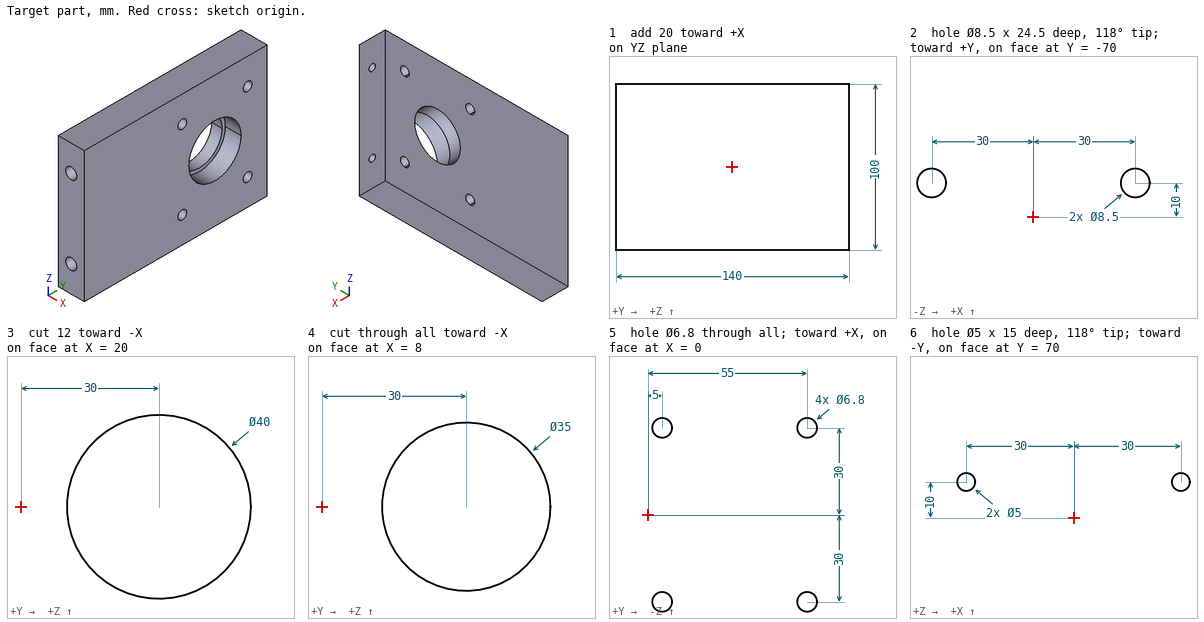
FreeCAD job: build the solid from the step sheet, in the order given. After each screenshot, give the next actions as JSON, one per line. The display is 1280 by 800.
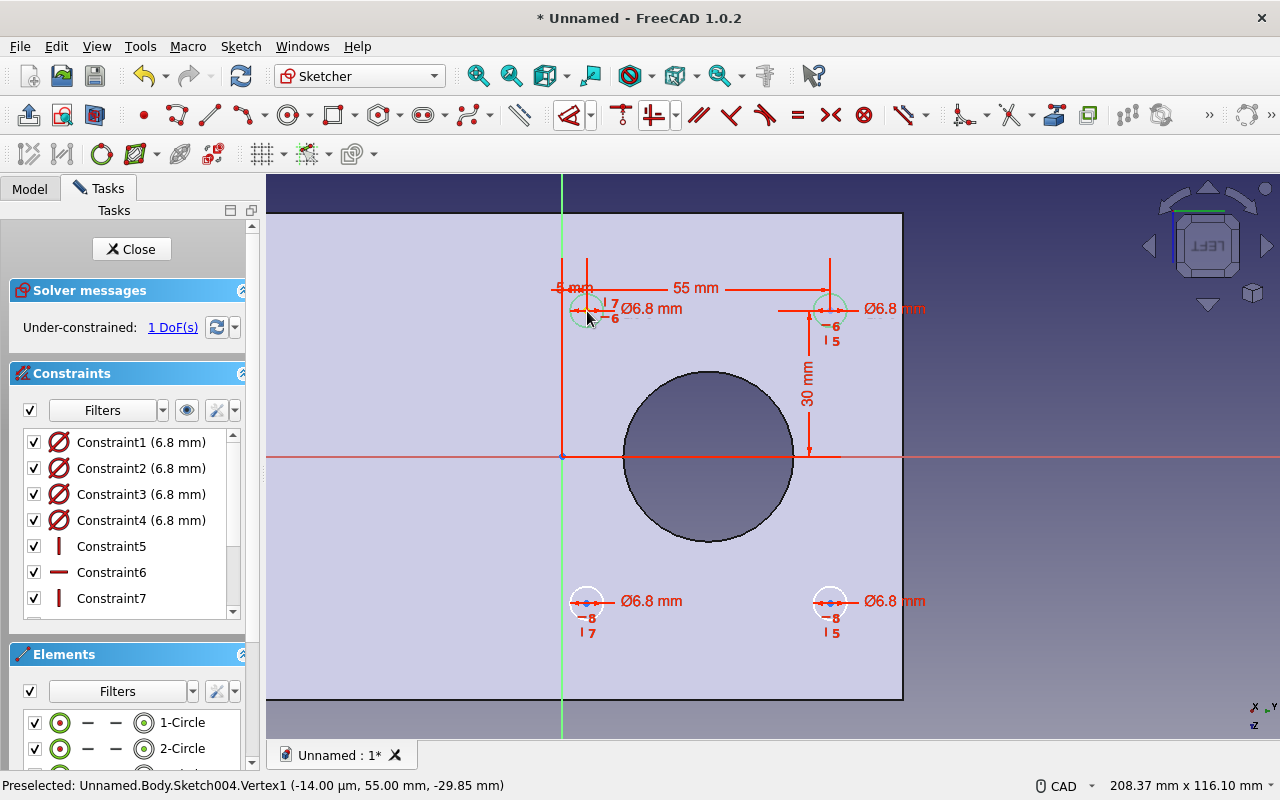
{"action": "left_click", "coordinate": [830, 603]}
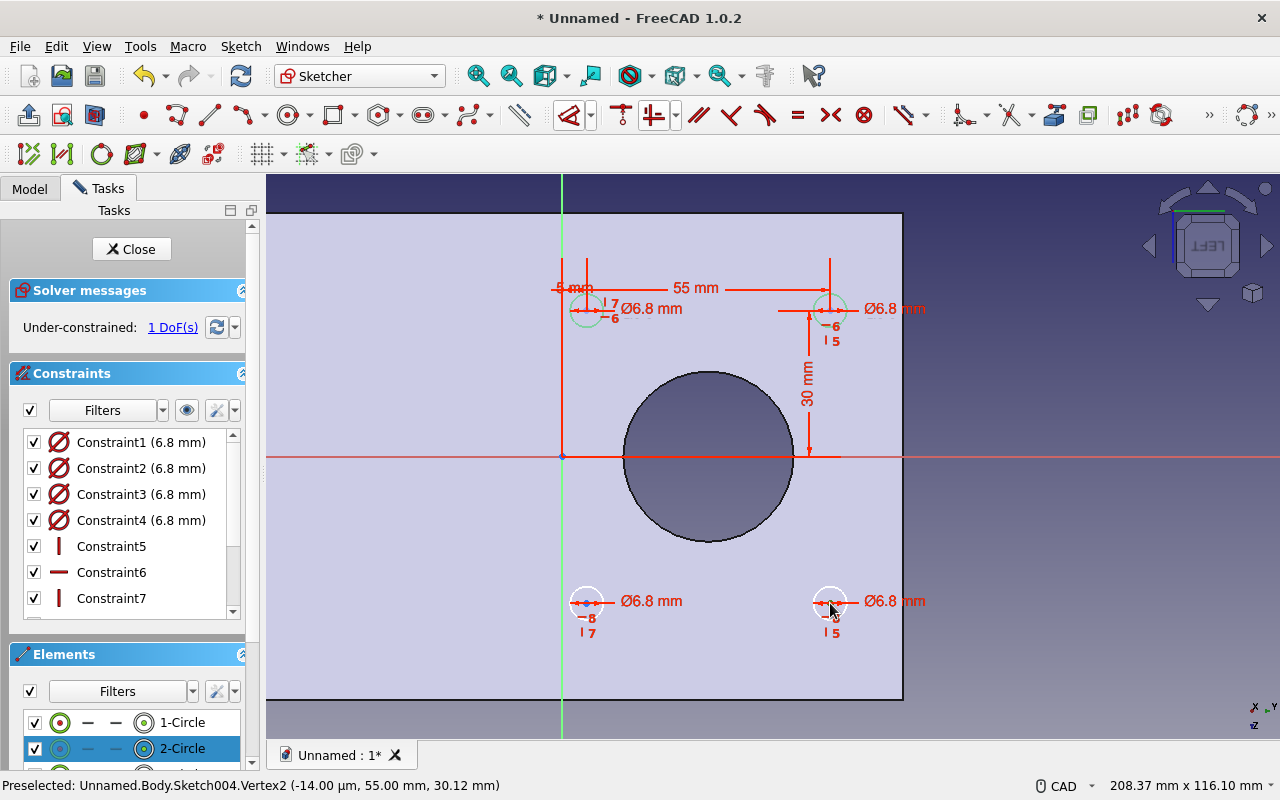
{"action": "key", "text": "i"}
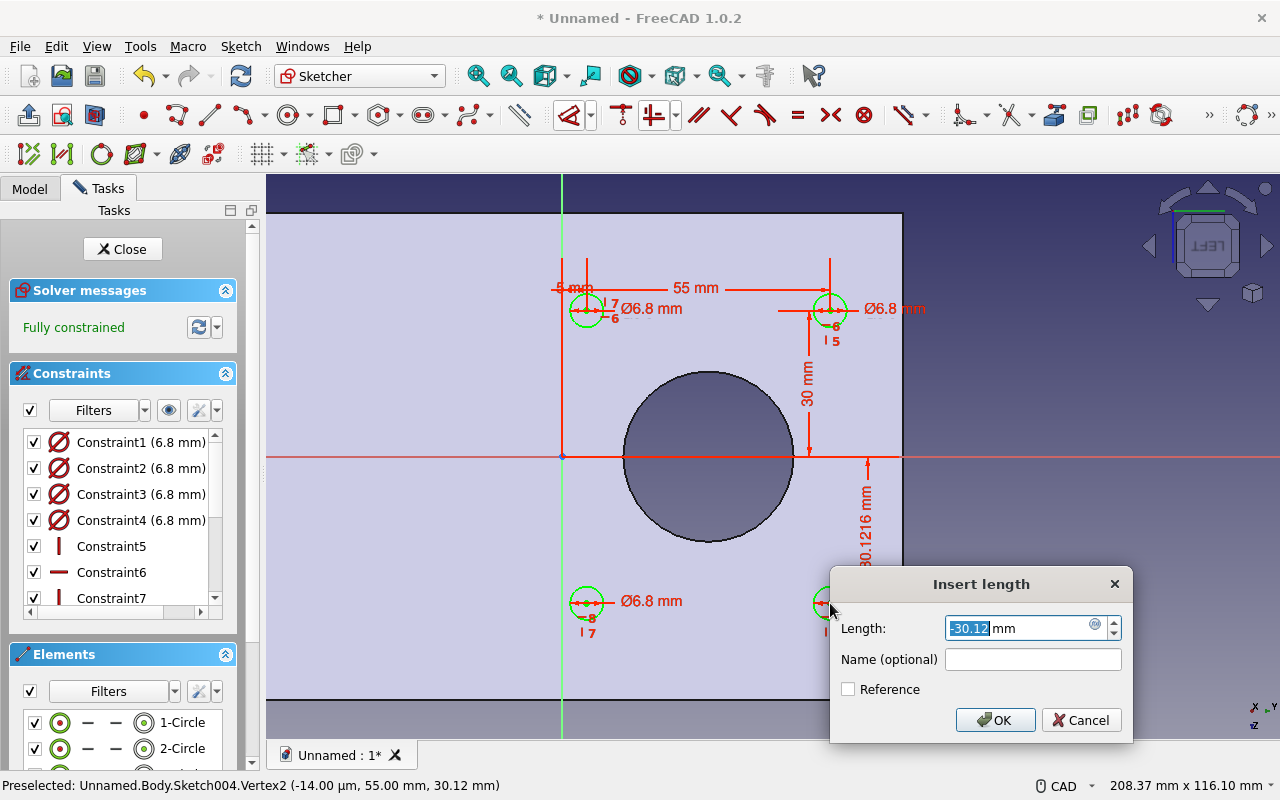
{"action": "type", "text": "-30"}
{"action": "key", "text": "Return"}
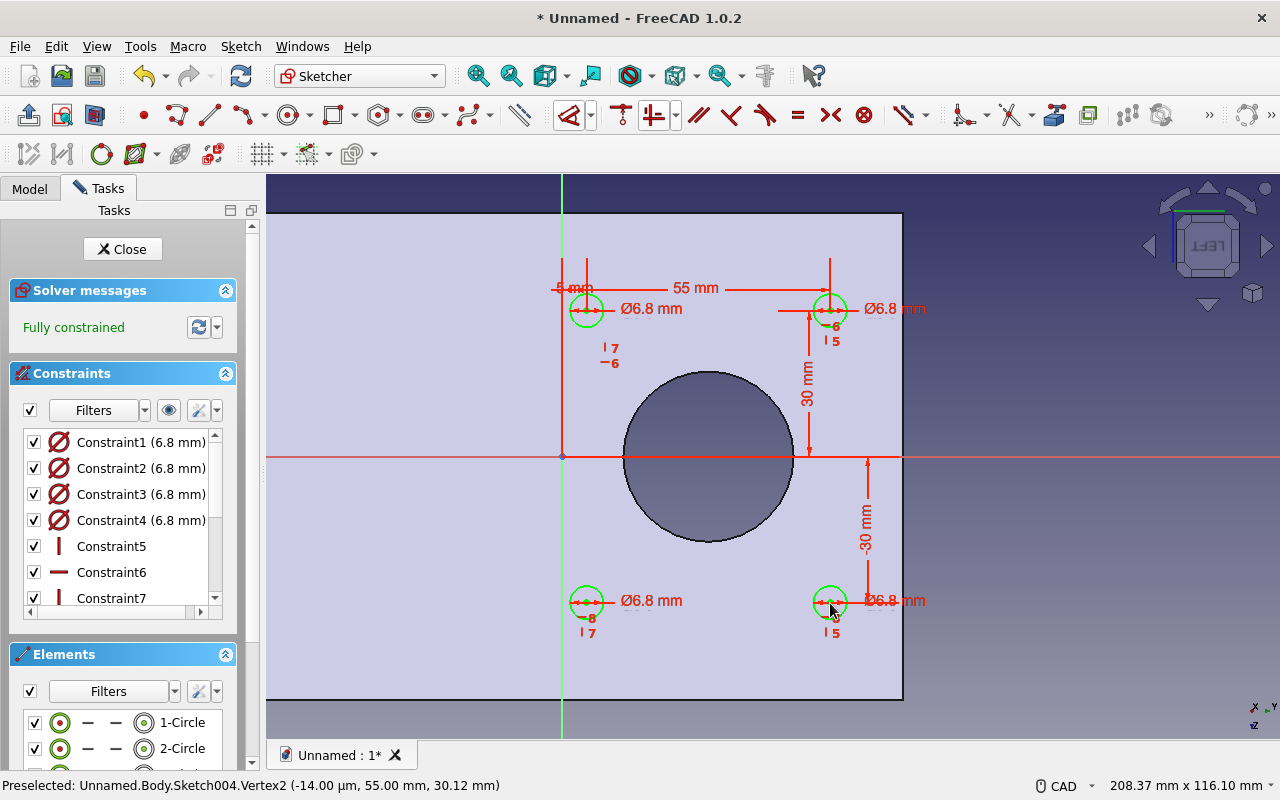
{"action": "left_click", "coordinate": [123, 249]}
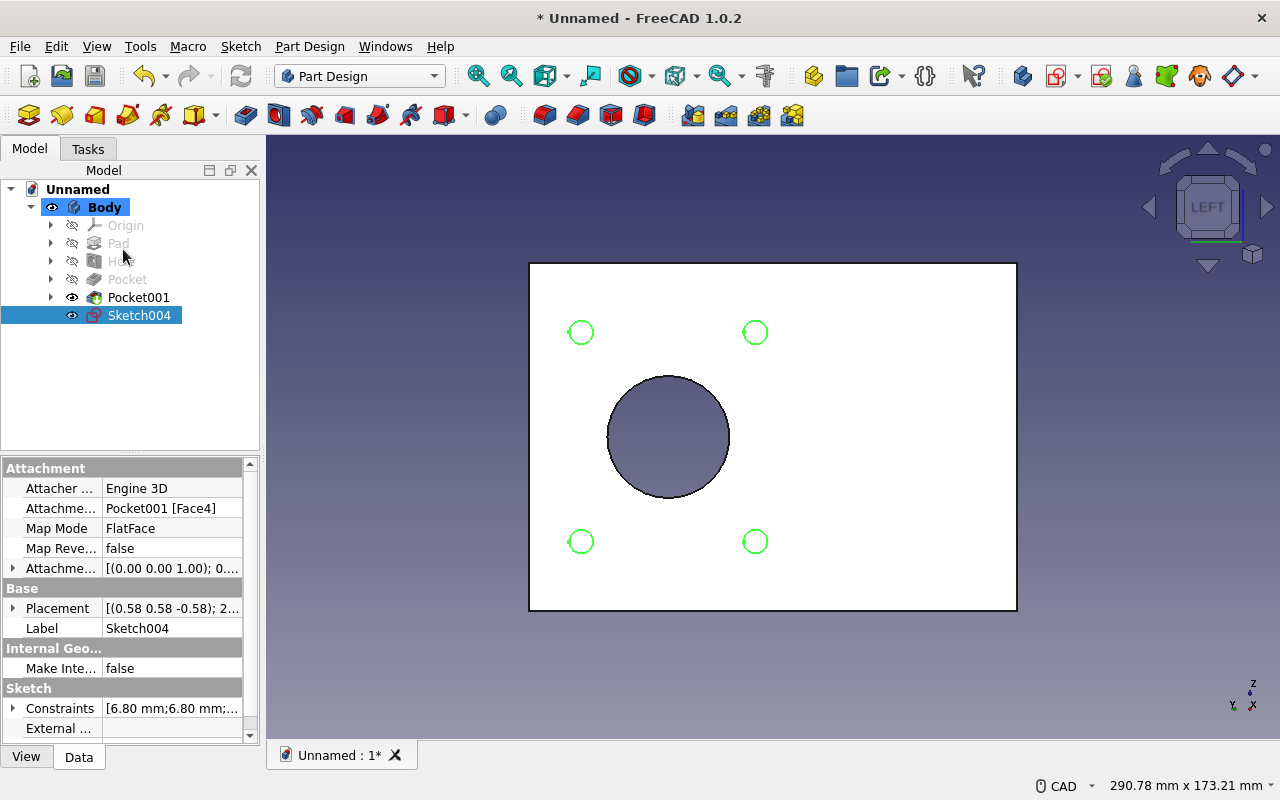
{"action": "left_click", "coordinate": [279, 116]}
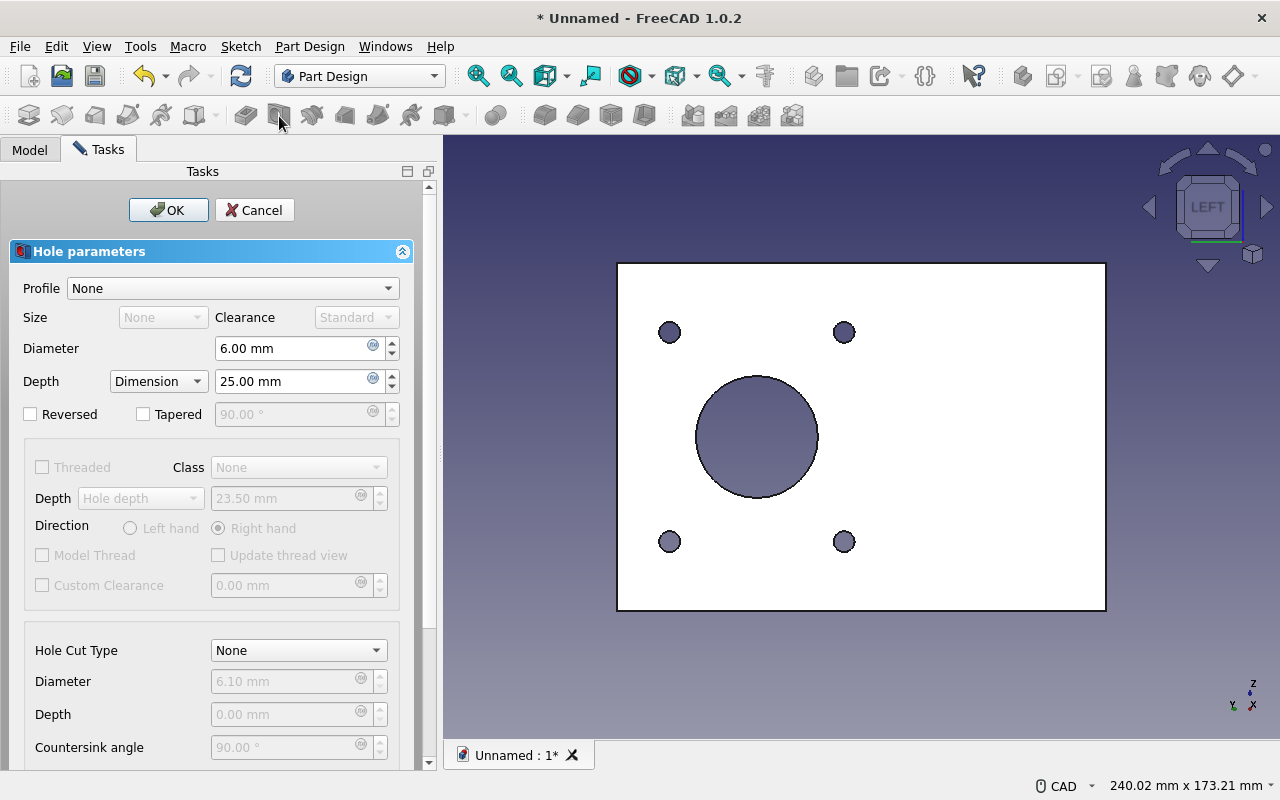
{"action": "triple_click", "coordinate": [300, 348]}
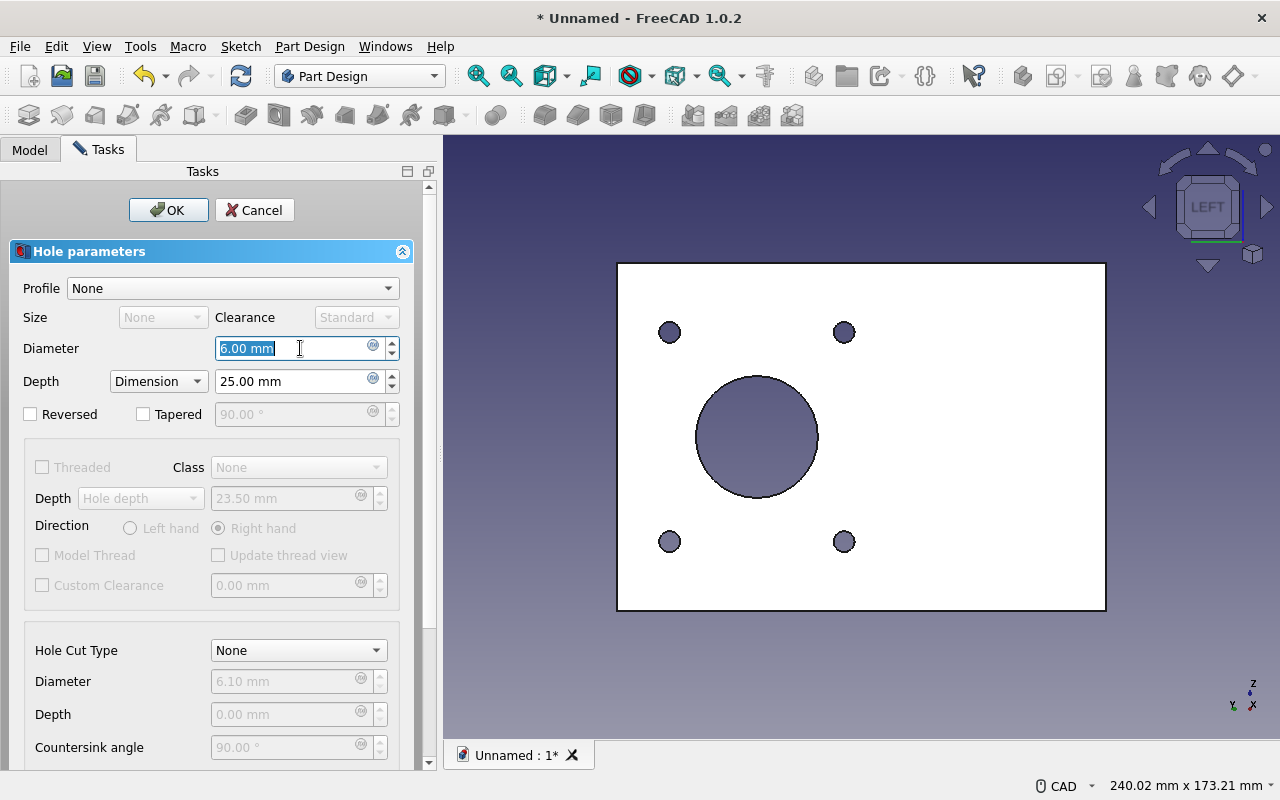
{"action": "type", "text": "6.8"}
{"action": "key", "text": "Tab"}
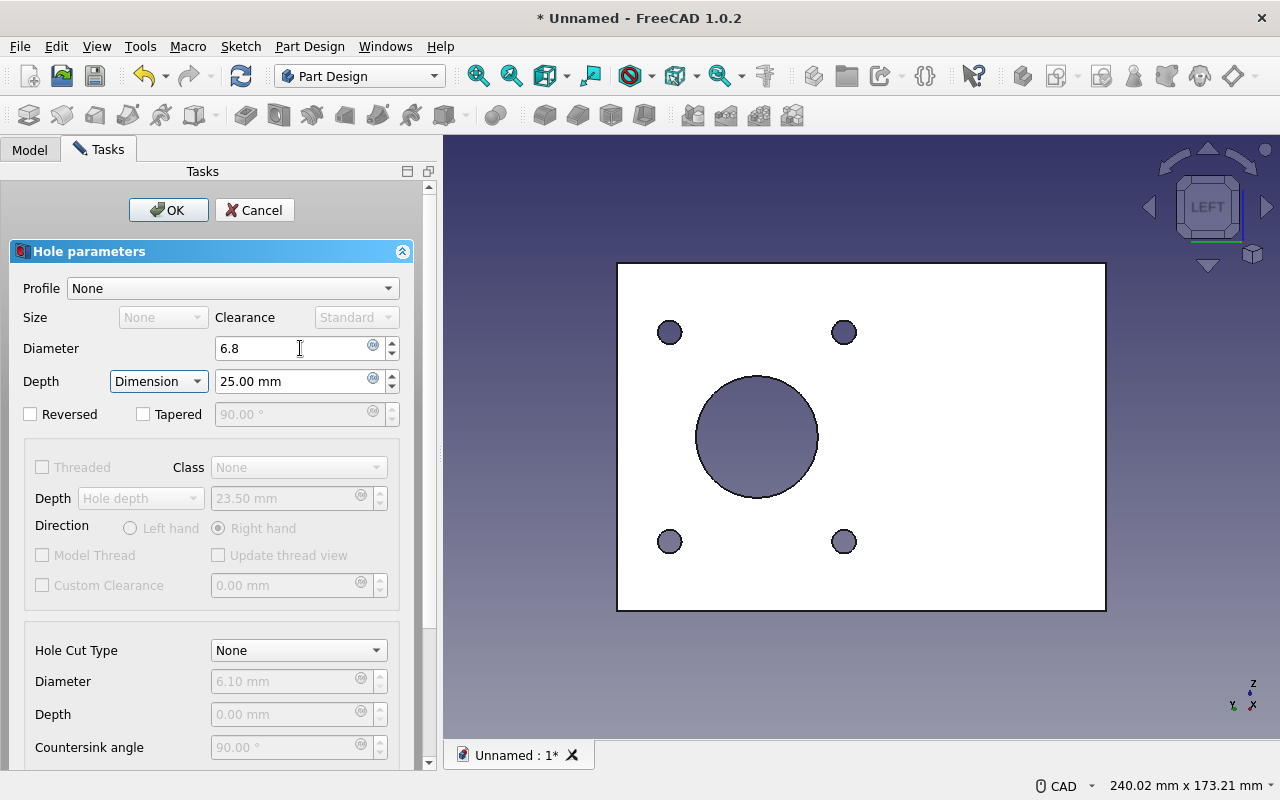
{"action": "left_click", "coordinate": [160, 382]}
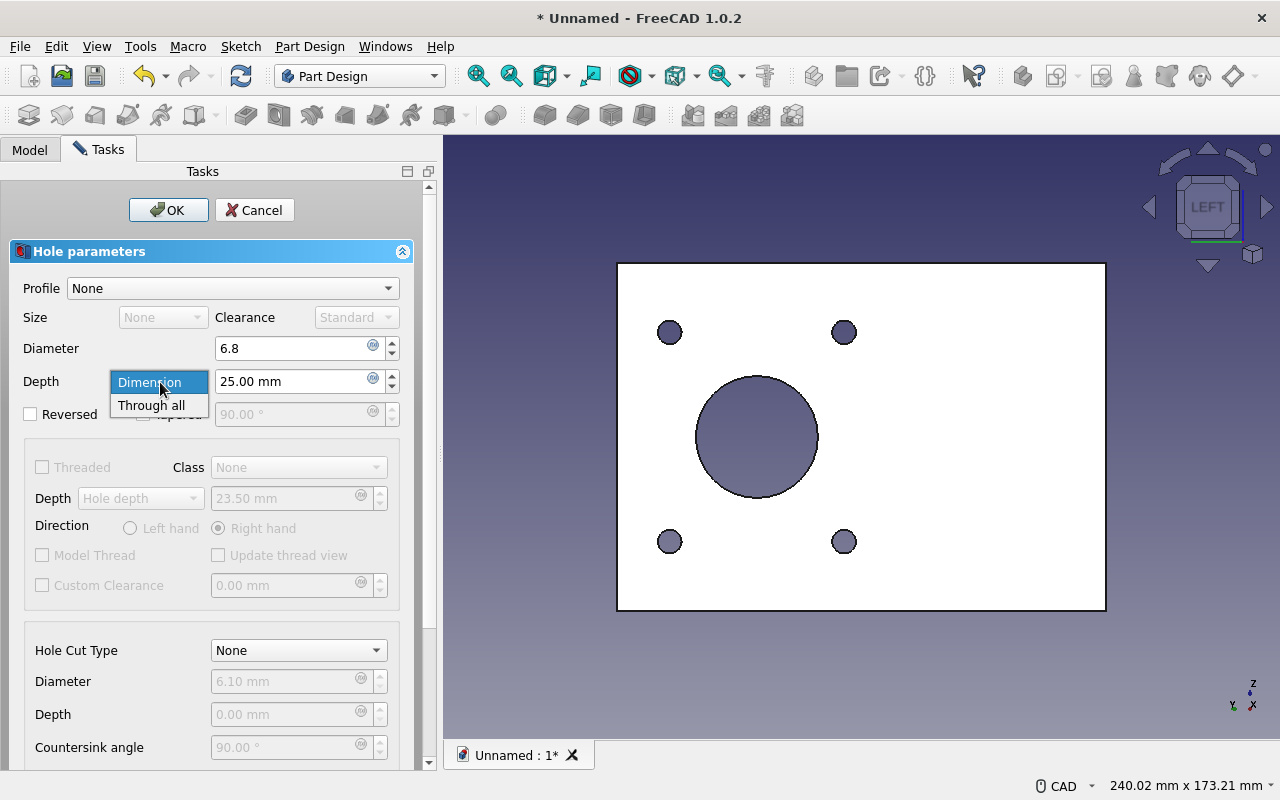
{"action": "left_click", "coordinate": [158, 406]}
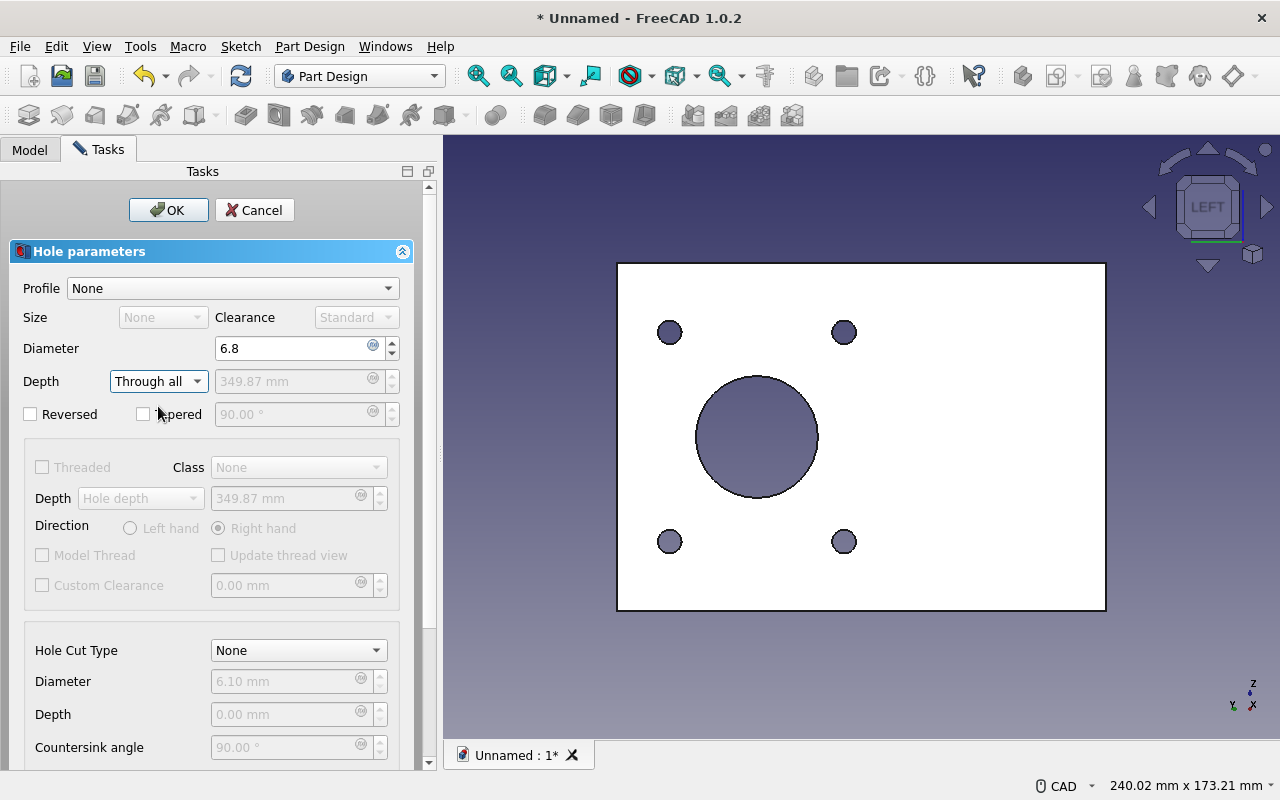
{"action": "left_click", "coordinate": [169, 210]}